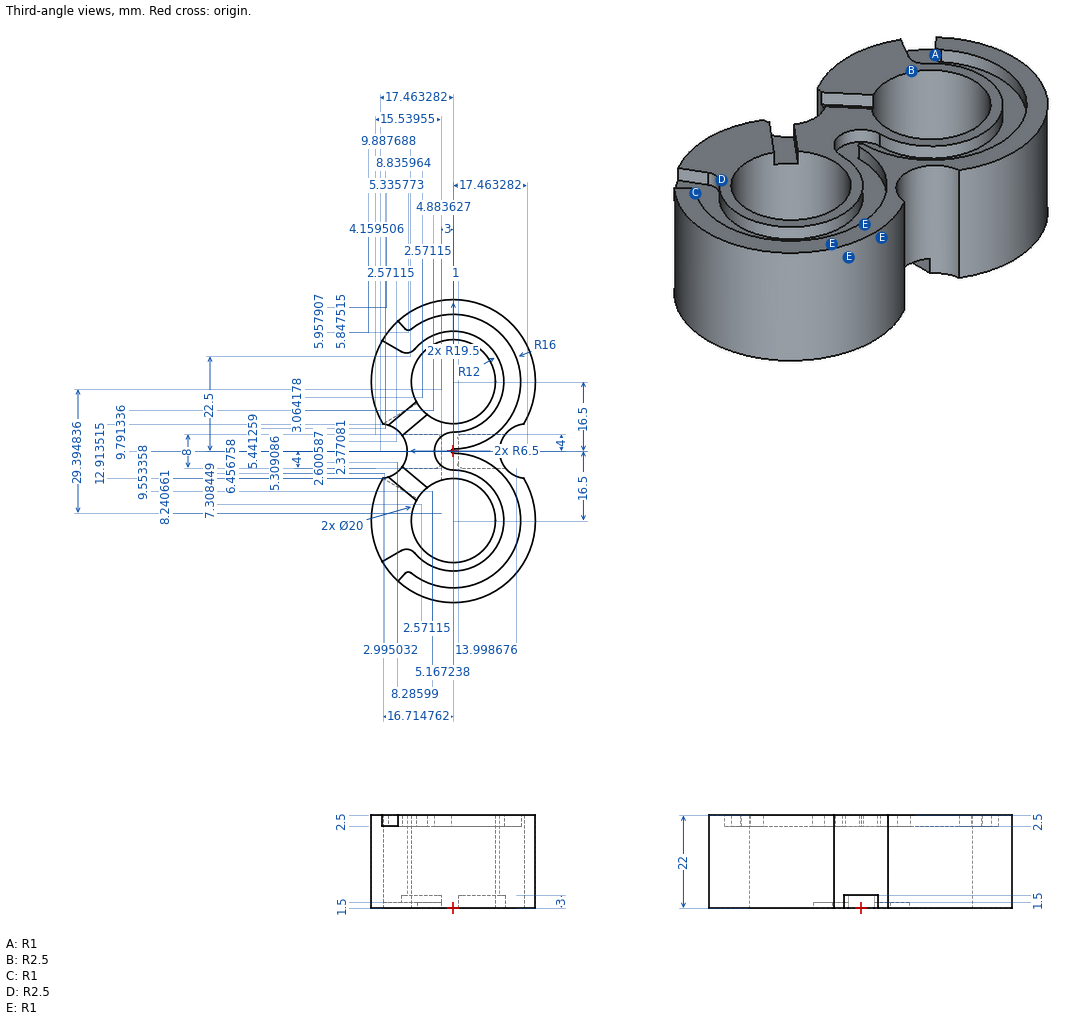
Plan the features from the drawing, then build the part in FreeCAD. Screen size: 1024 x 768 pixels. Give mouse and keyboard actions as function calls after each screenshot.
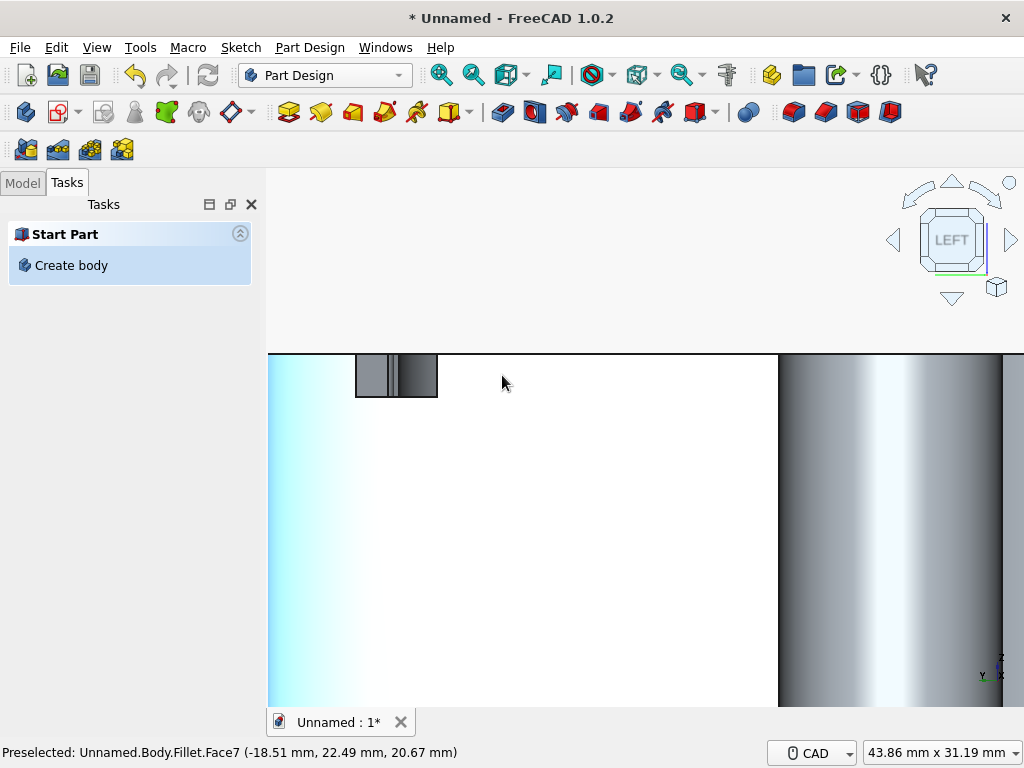
key(v)
key(f)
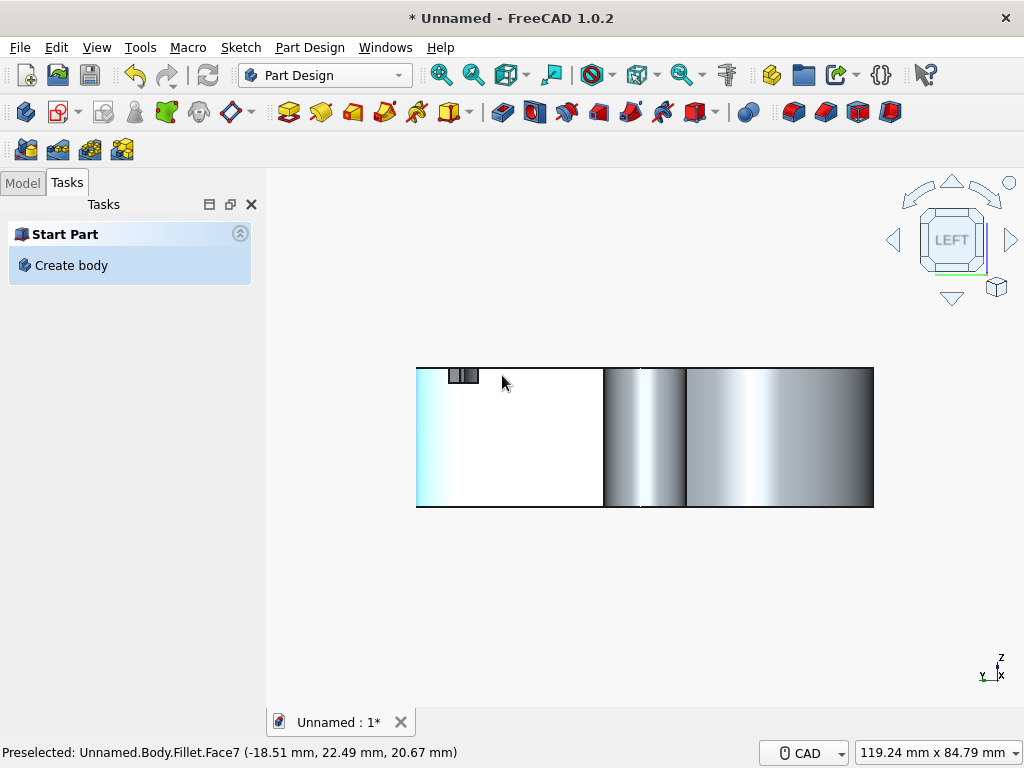
key(v)
key(3)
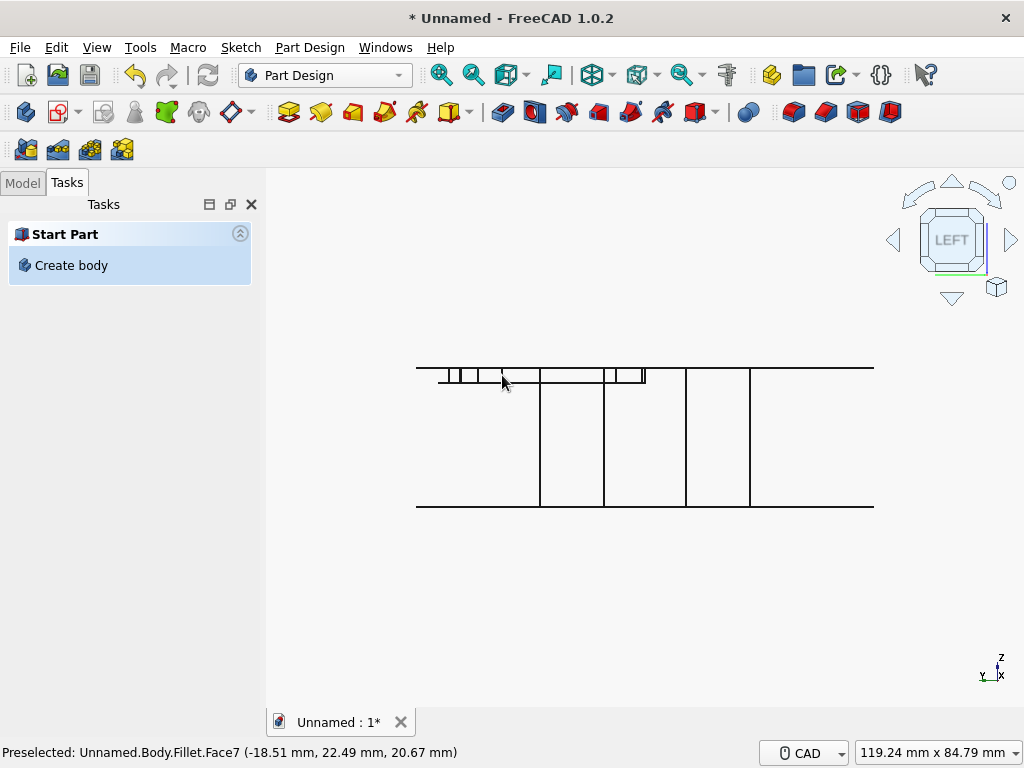
key(0)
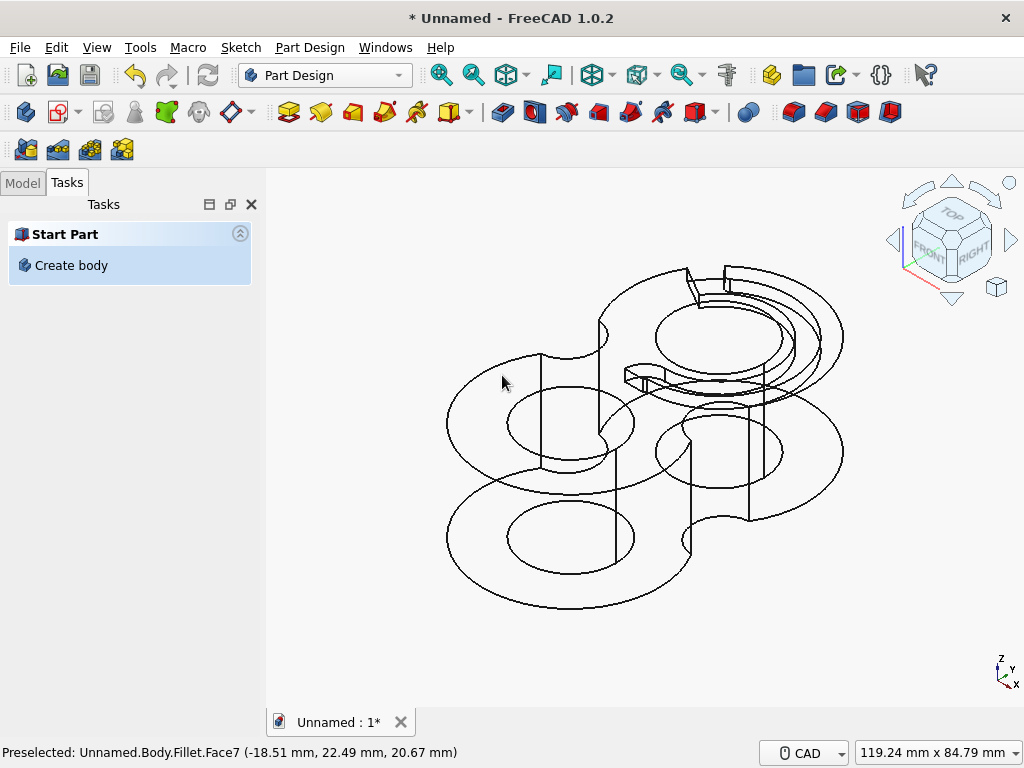
scroll(699, 301, up, 6)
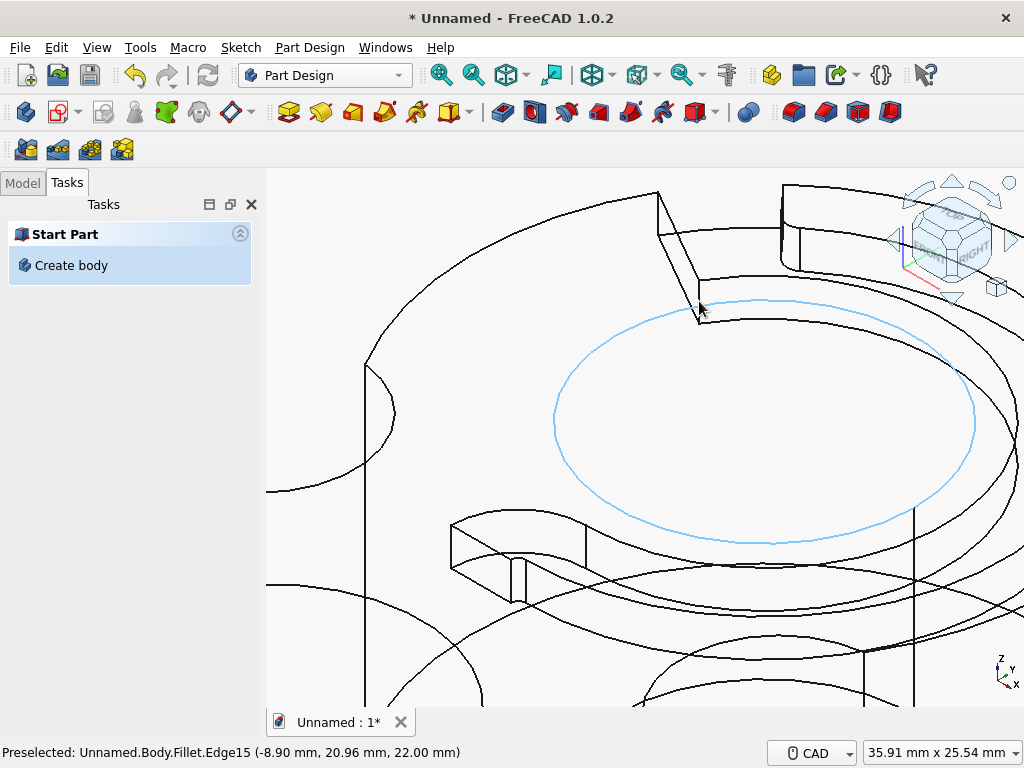
click(699, 297)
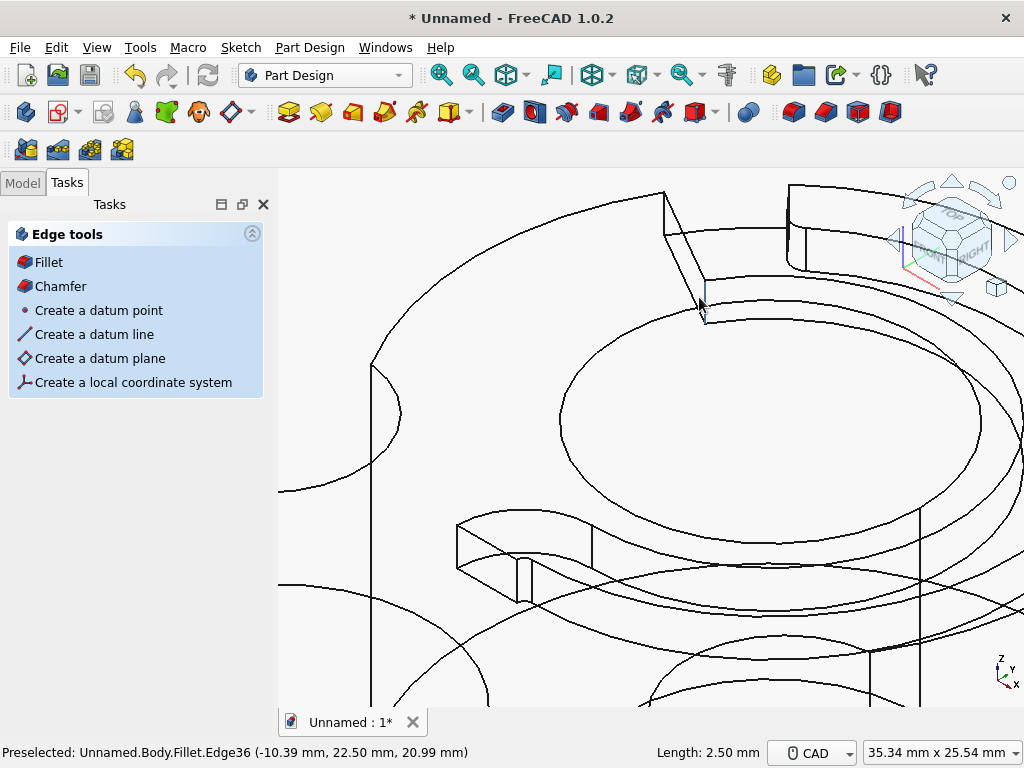
key(v)
key(1)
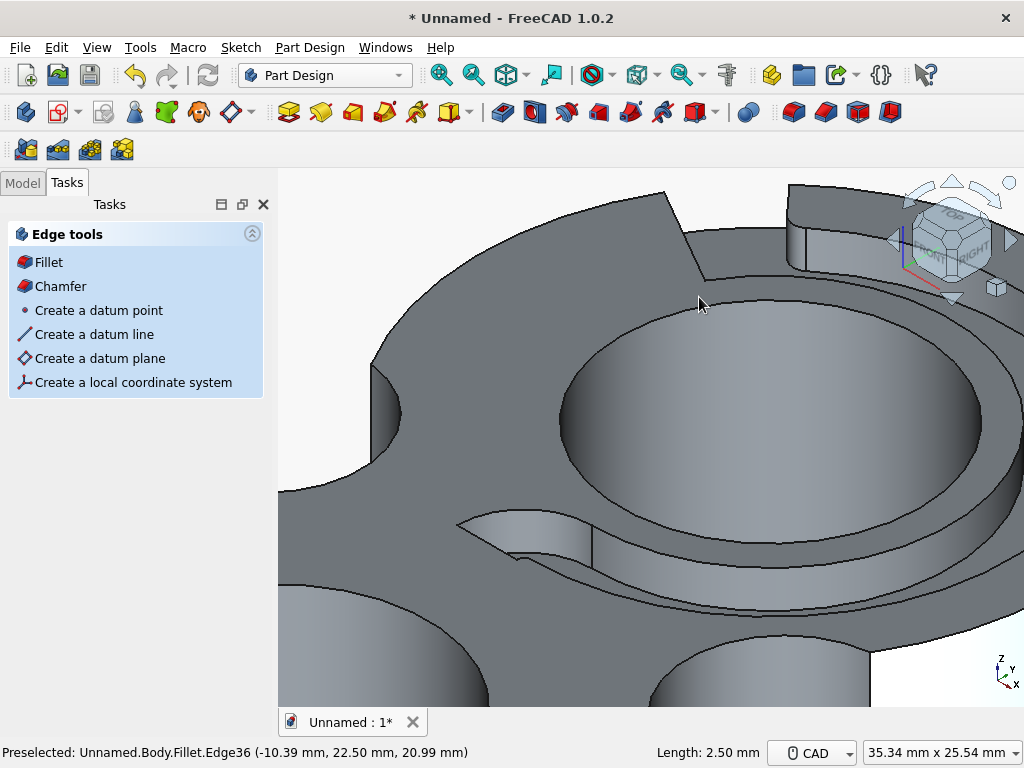
click(794, 112)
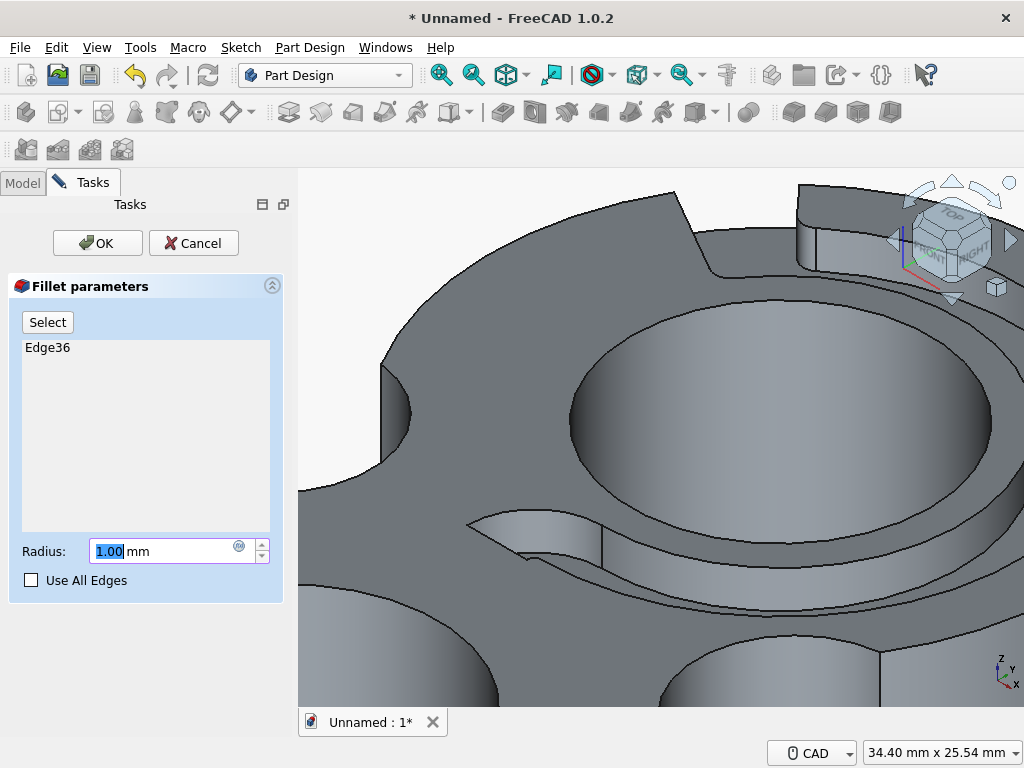
text(2.5)
key(Tab)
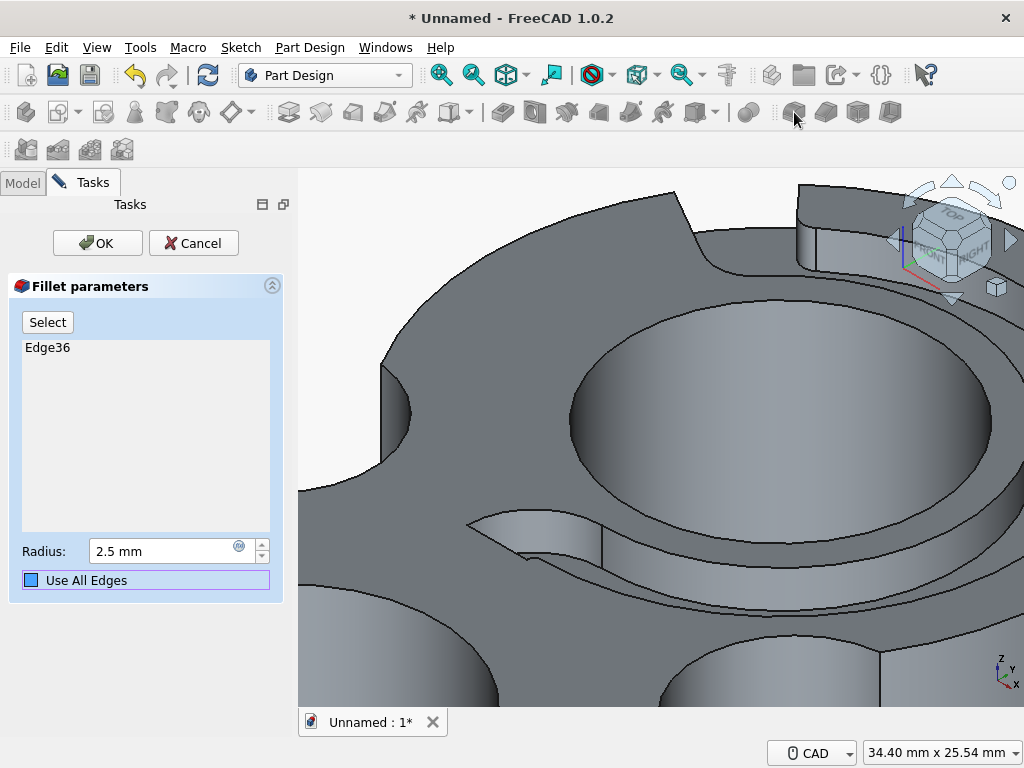
click(98, 243)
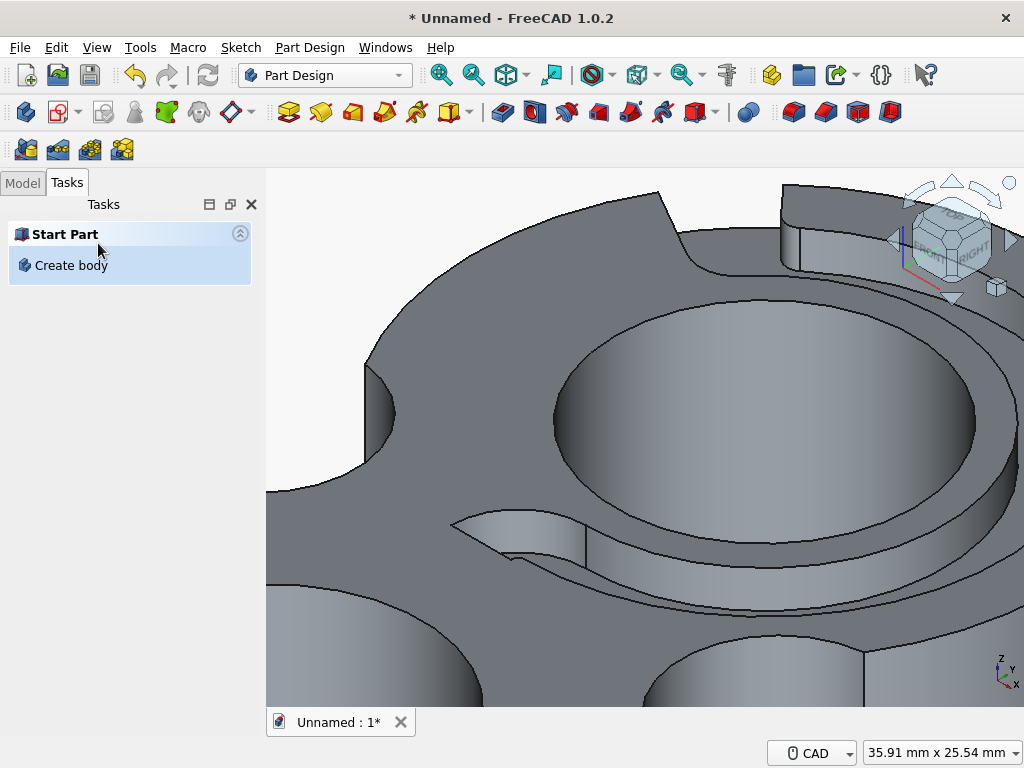
key(v)
key(f)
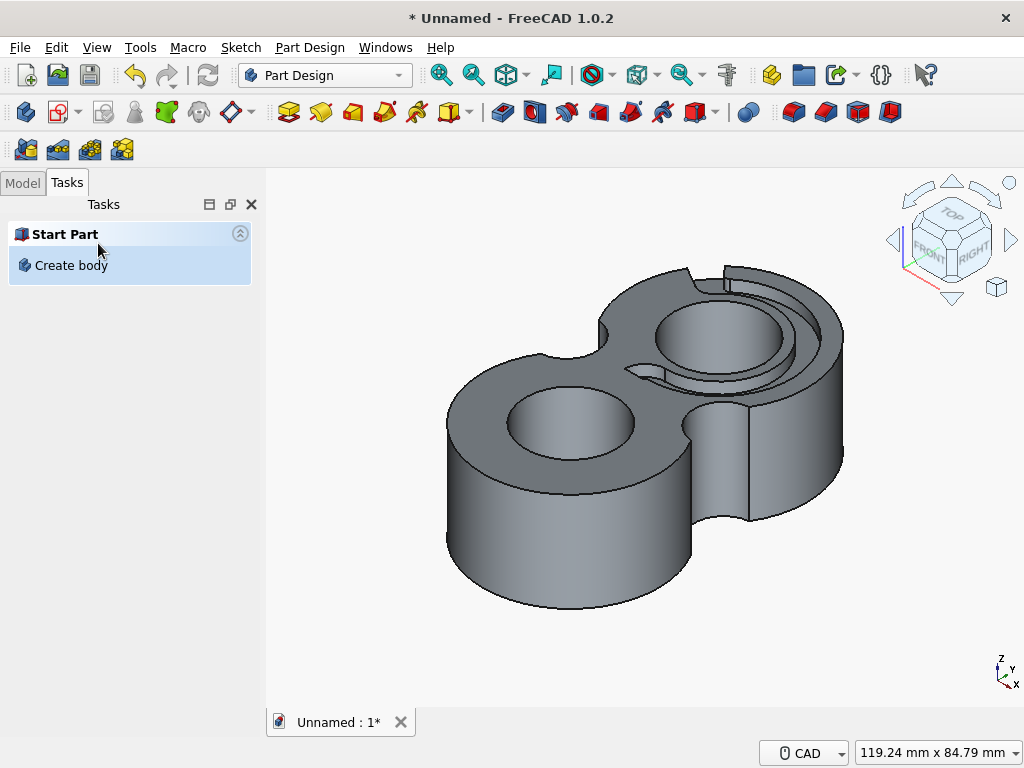
click(23, 182)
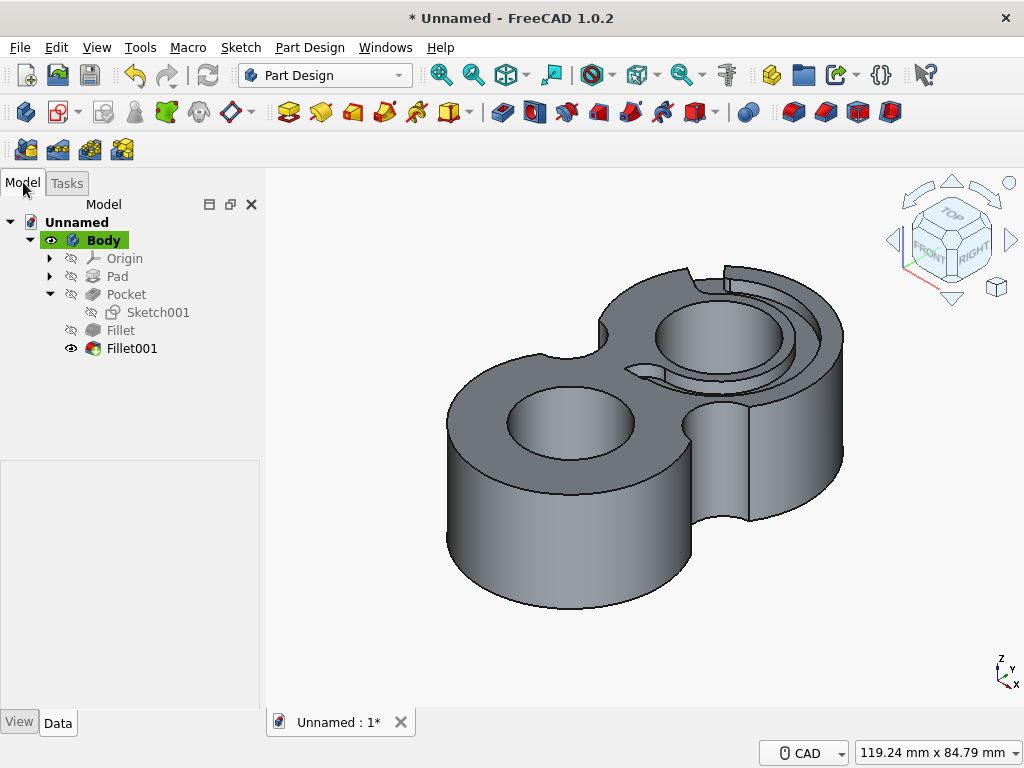
click(116, 294)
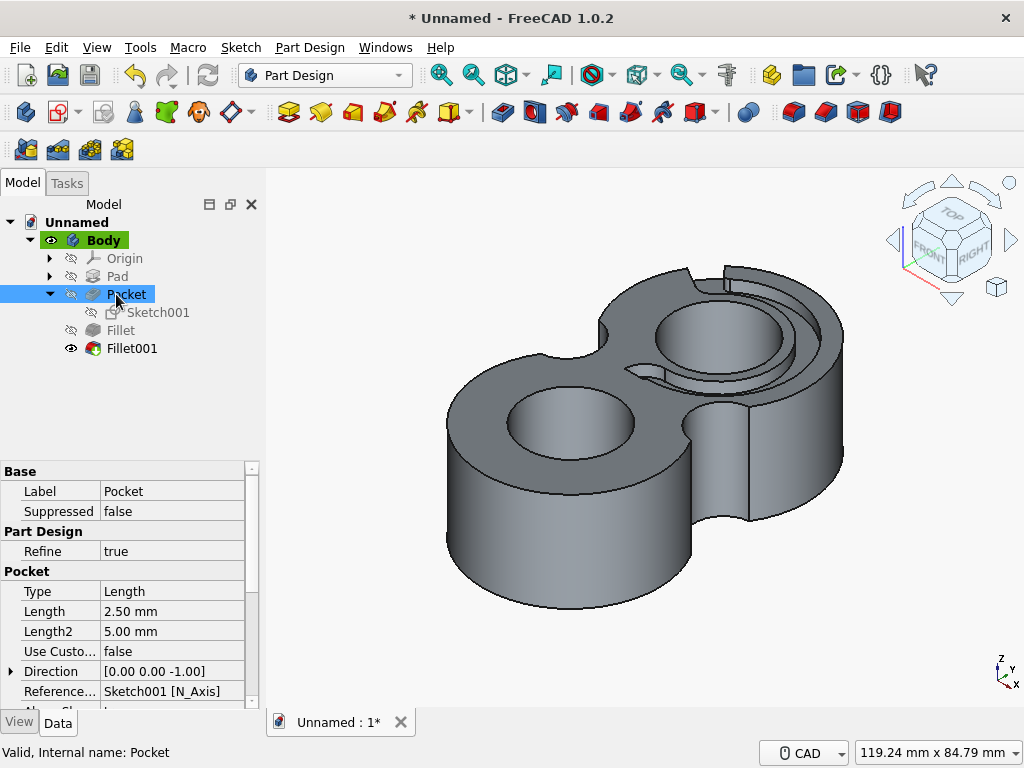
click(26, 150)